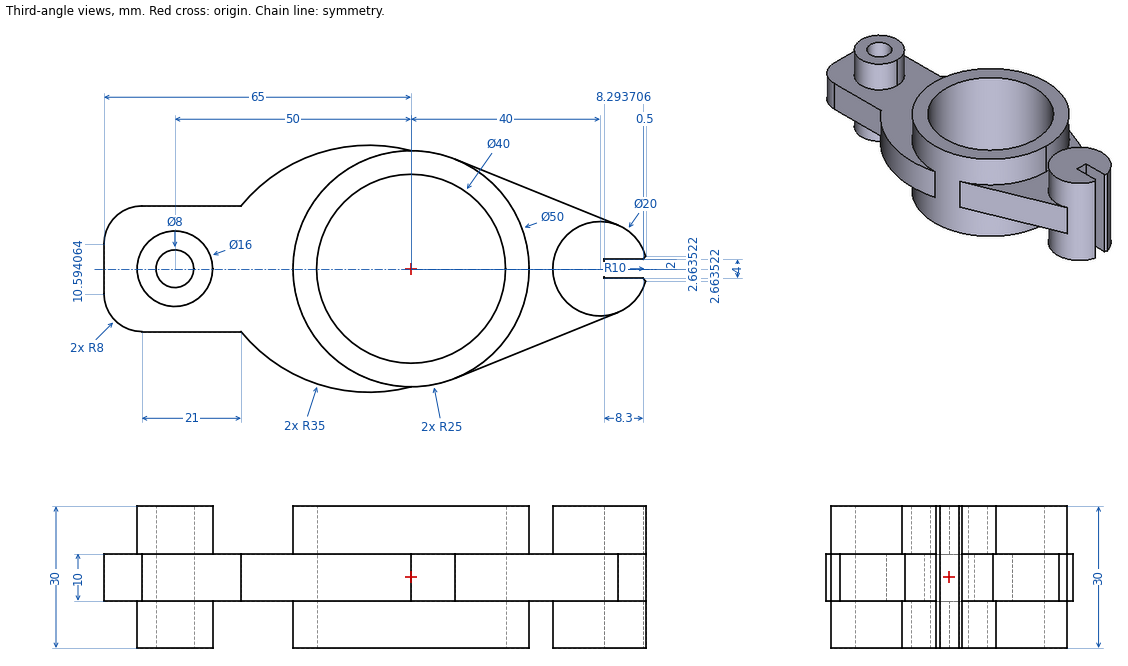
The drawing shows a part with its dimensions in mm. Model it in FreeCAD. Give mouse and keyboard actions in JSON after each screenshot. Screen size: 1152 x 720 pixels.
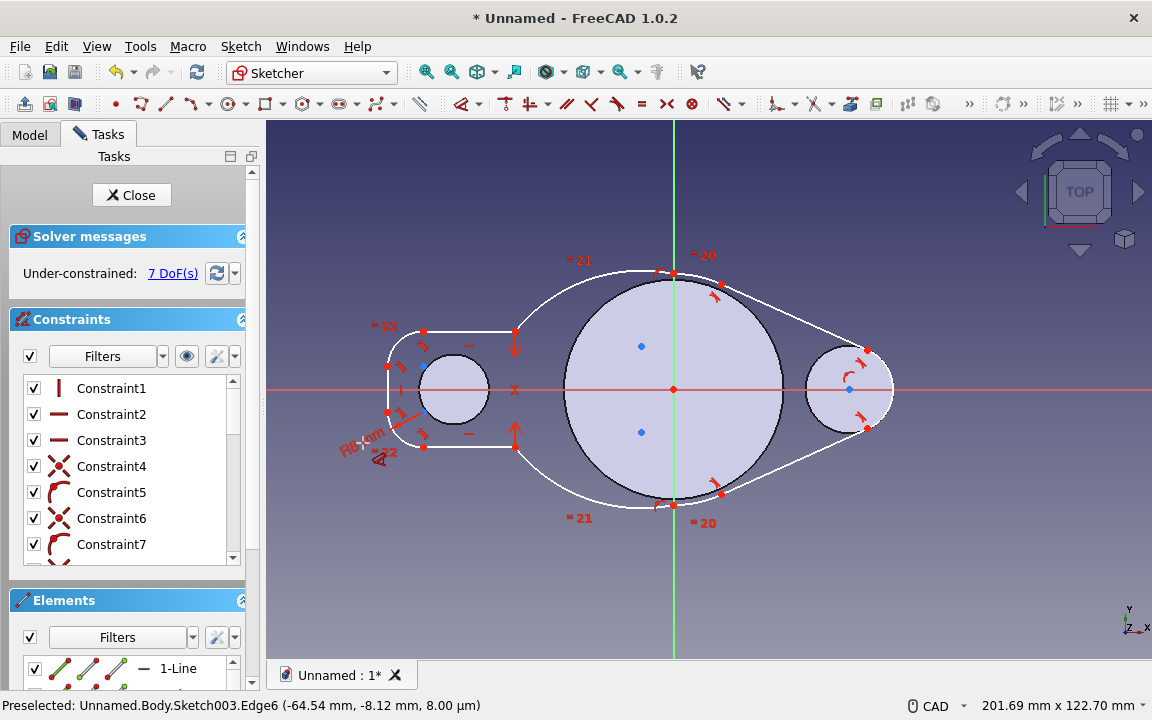
{"action": "left_click", "coordinate": [555, 483]}
{"action": "left_click", "coordinate": [538, 510]}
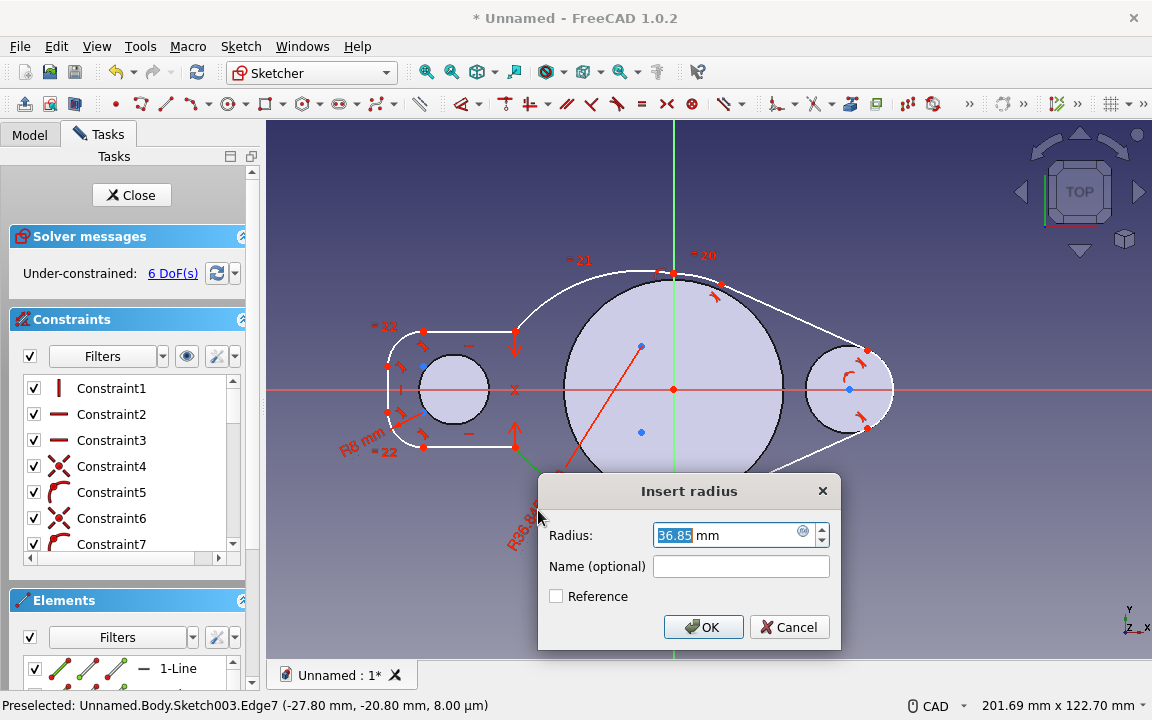
{"action": "type", "text": "35"}
{"action": "key", "text": "Return"}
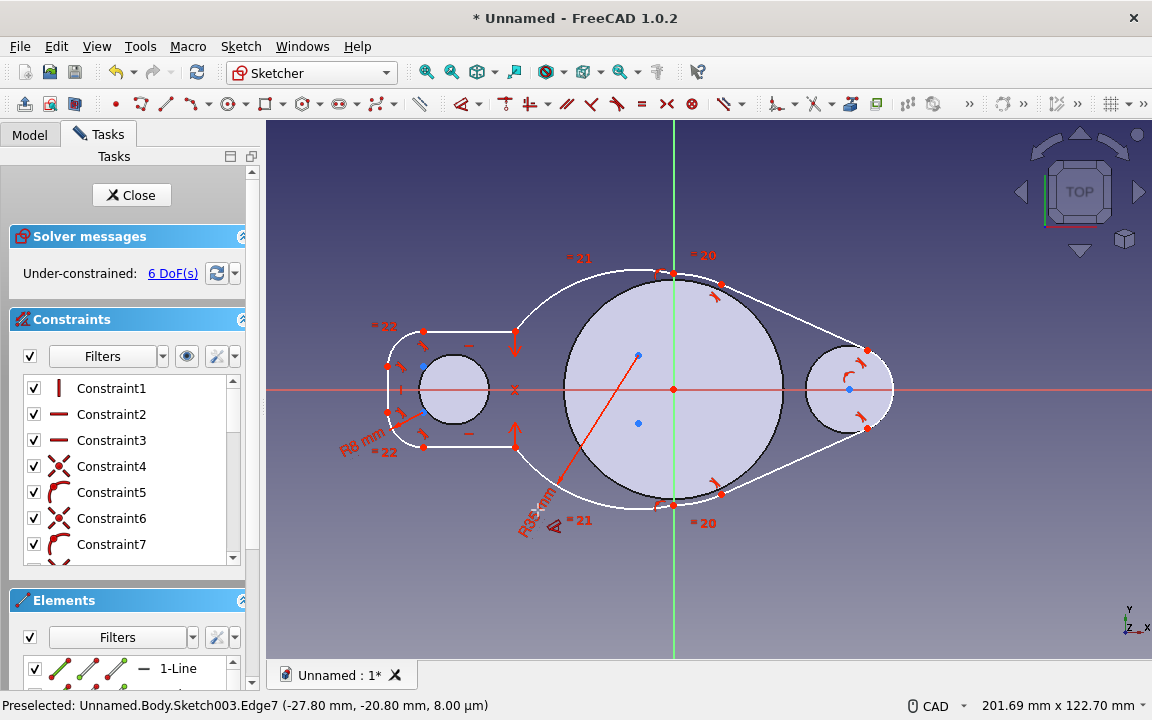
{"action": "left_click", "coordinate": [688, 504]}
{"action": "left_click", "coordinate": [692, 536]}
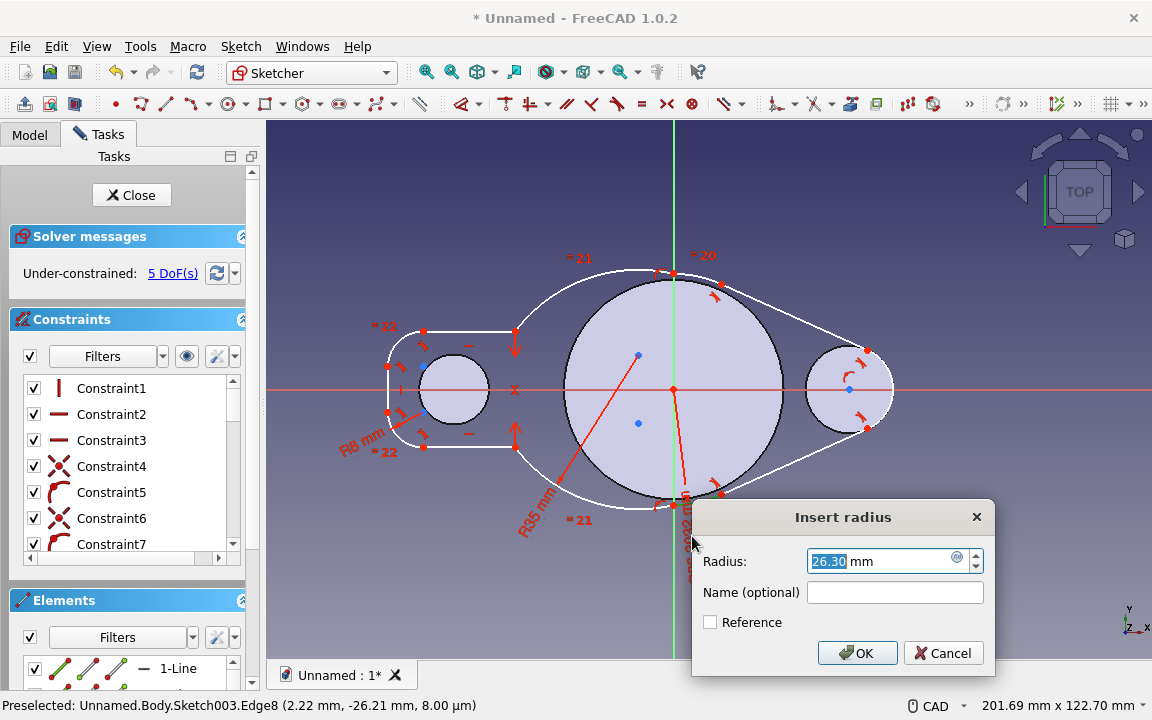
{"action": "type", "text": "25"}
{"action": "key", "text": "Return"}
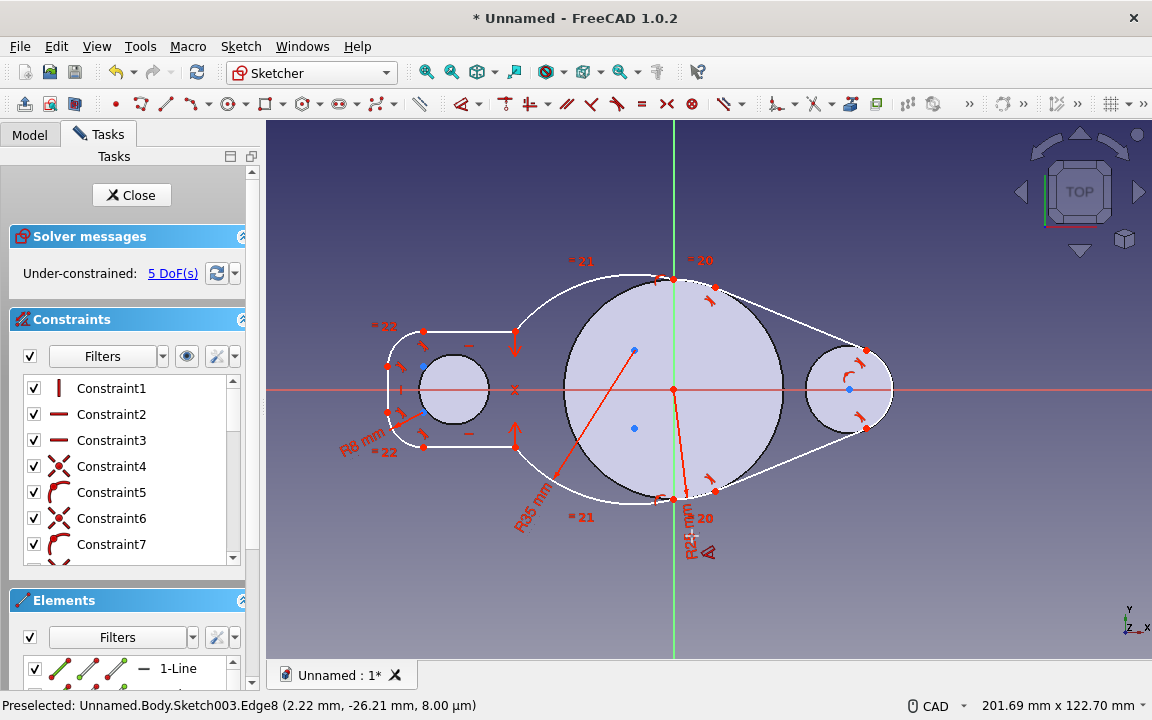
{"action": "left_click", "coordinate": [888, 409]}
{"action": "left_click", "coordinate": [917, 424]}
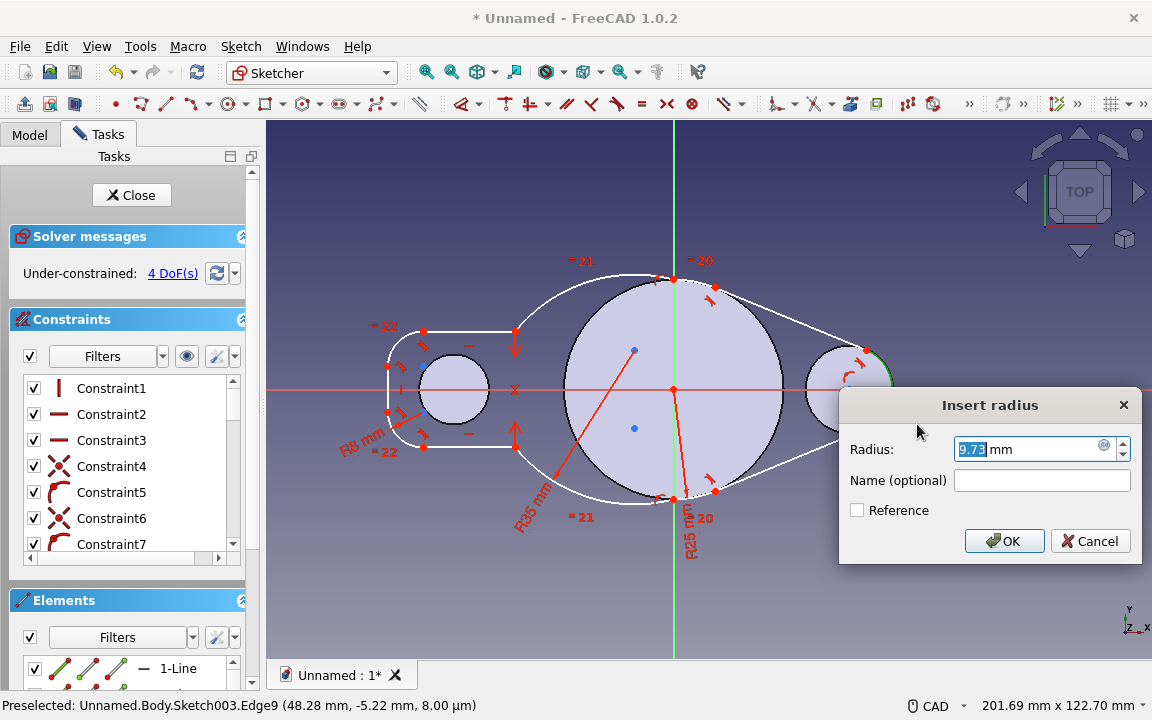
{"action": "type", "text": "10"}
{"action": "key", "text": "Return"}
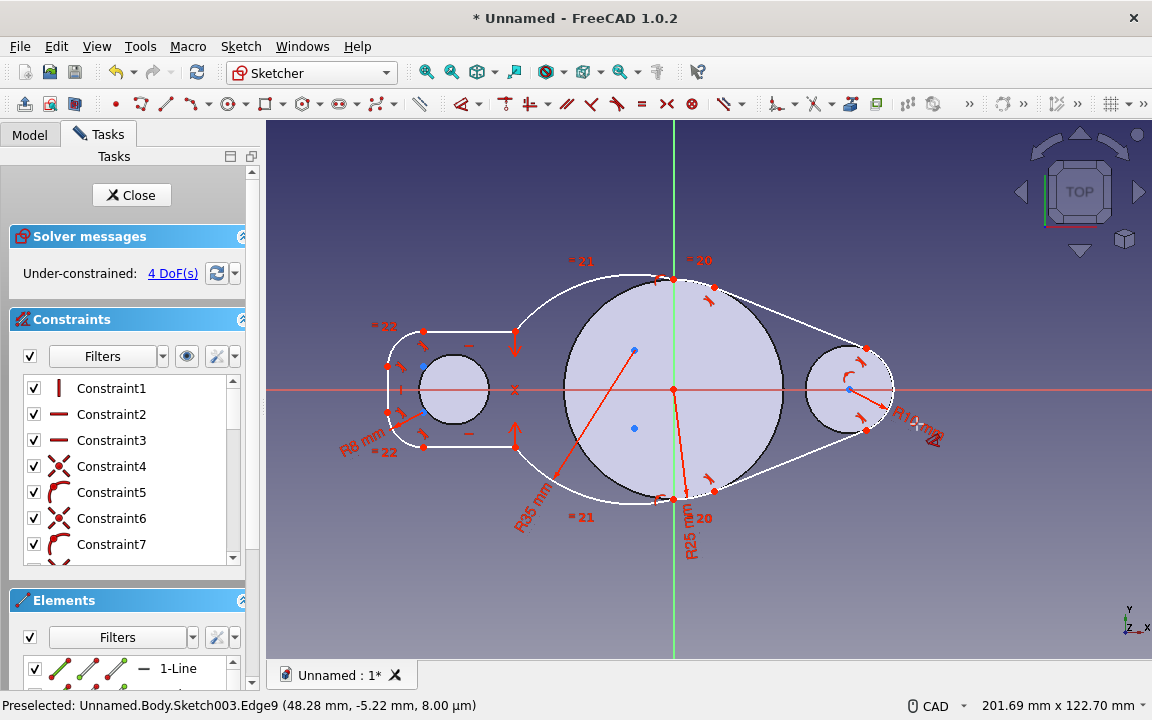
{"action": "left_click", "coordinate": [451, 447]}
{"action": "left_click", "coordinate": [469, 481]}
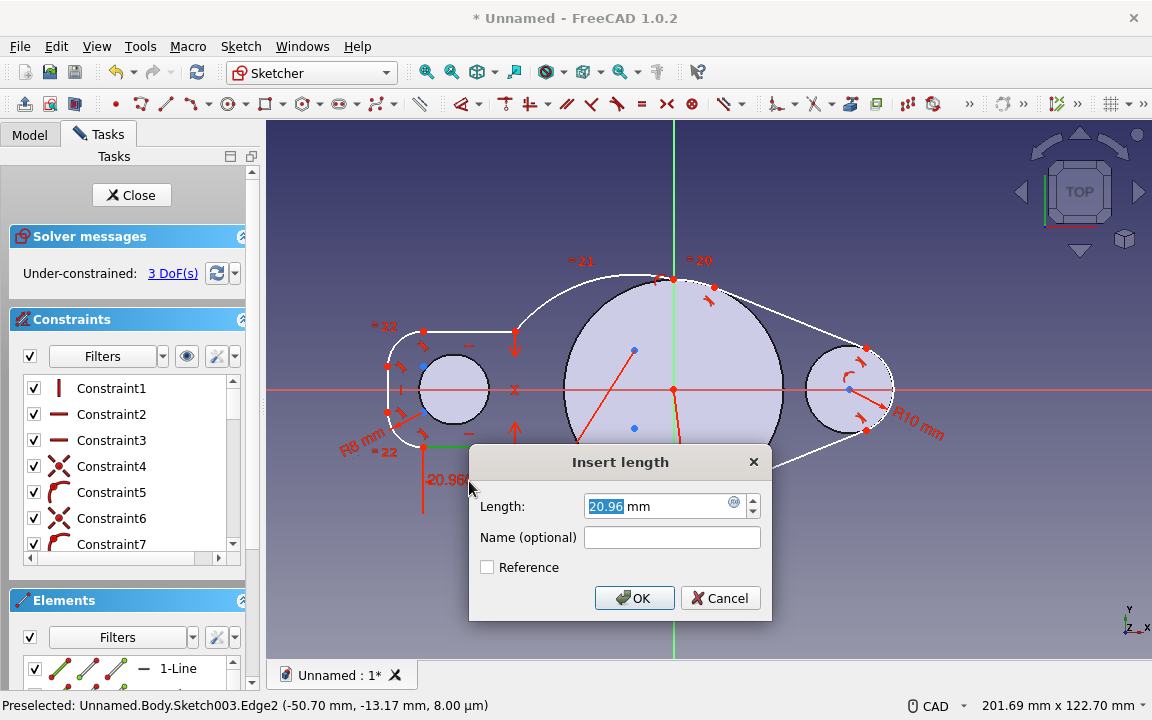
{"action": "type", "text": "21"}
{"action": "key", "text": "Return"}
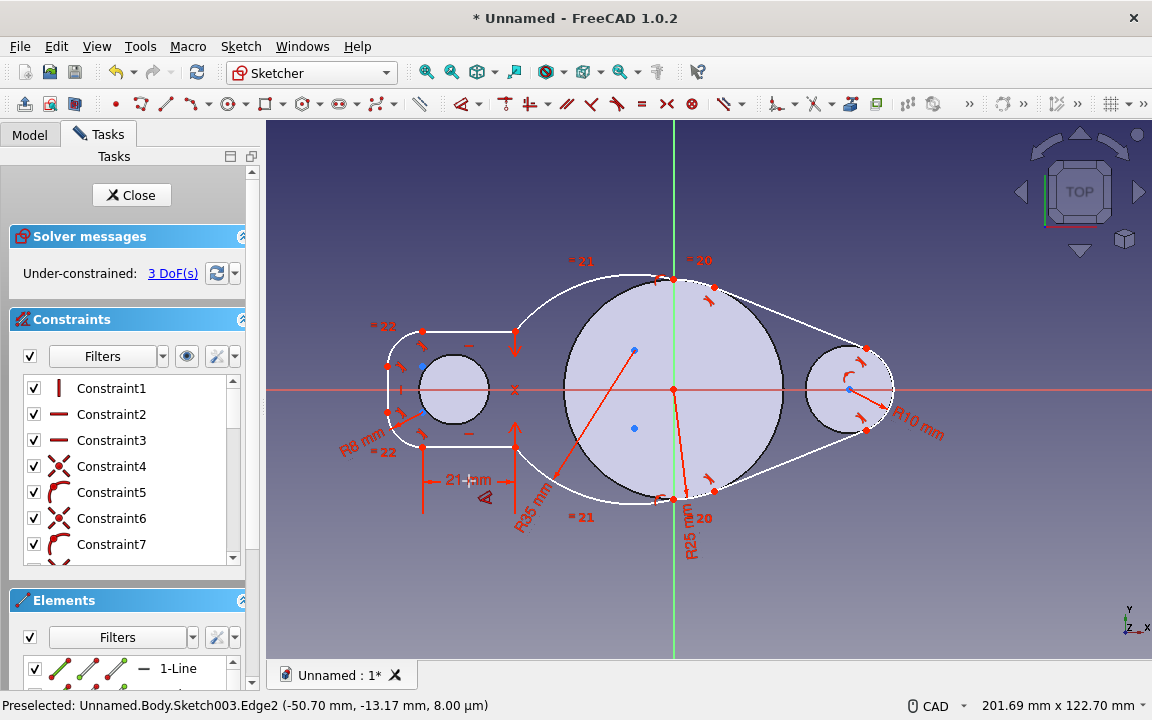
{"action": "left_click", "coordinate": [388, 367]}
{"action": "left_click", "coordinate": [597, 333]}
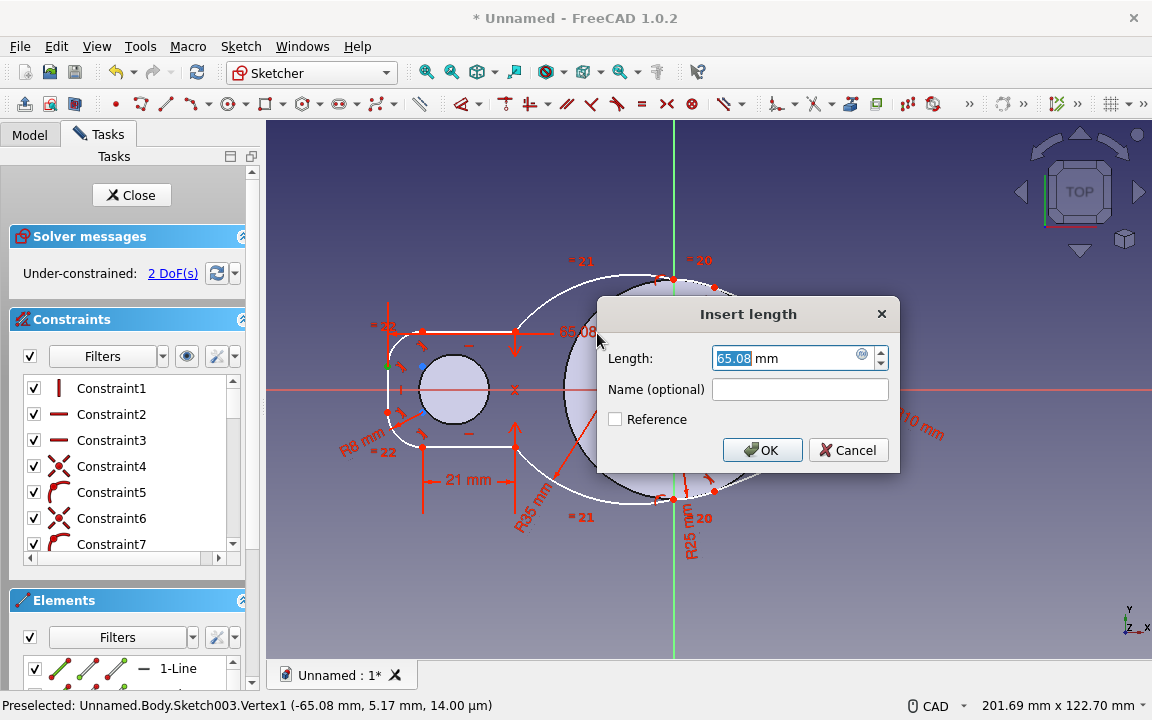
{"action": "type", "text": "65"}
{"action": "key", "text": "Return"}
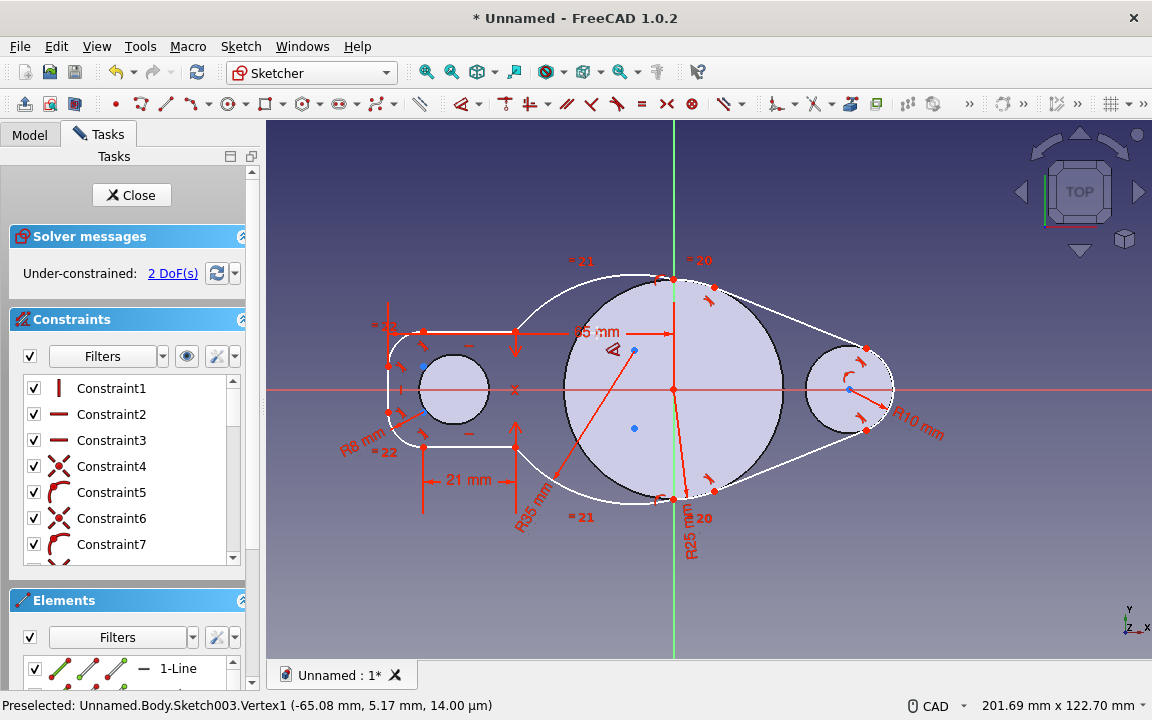
{"action": "left_click", "coordinate": [850, 390]}
{"action": "left_click", "coordinate": [762, 424]}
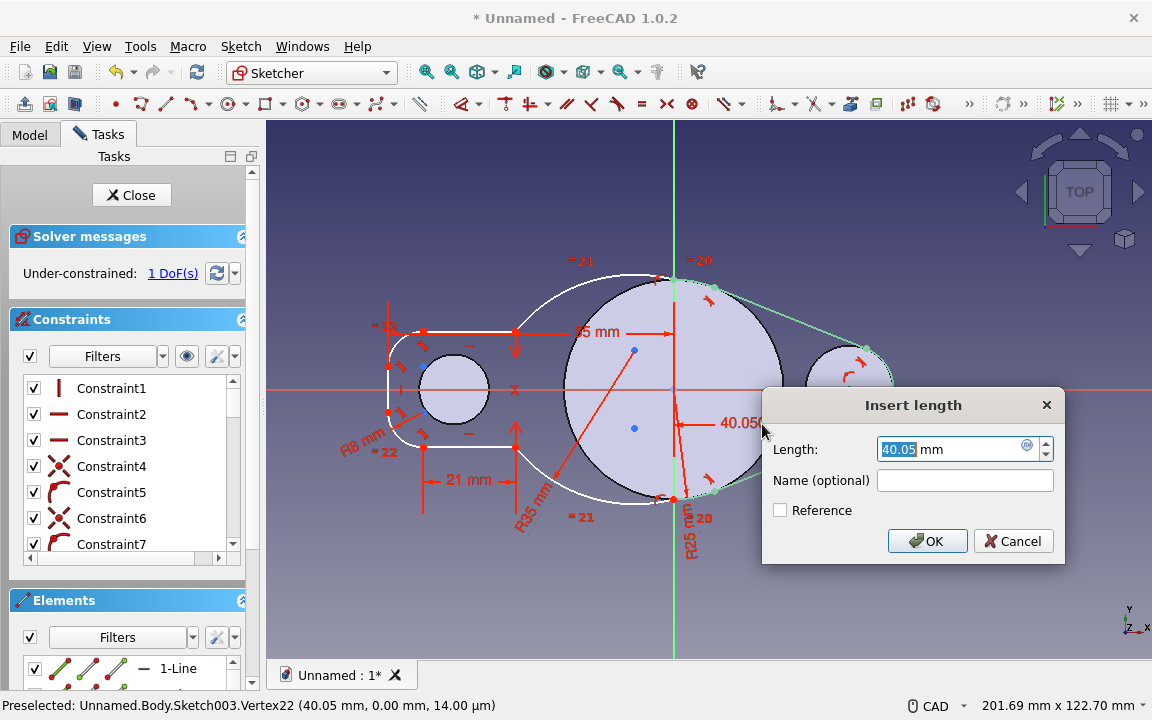
{"action": "type", "text": "40"}
{"action": "key", "text": "Return"}